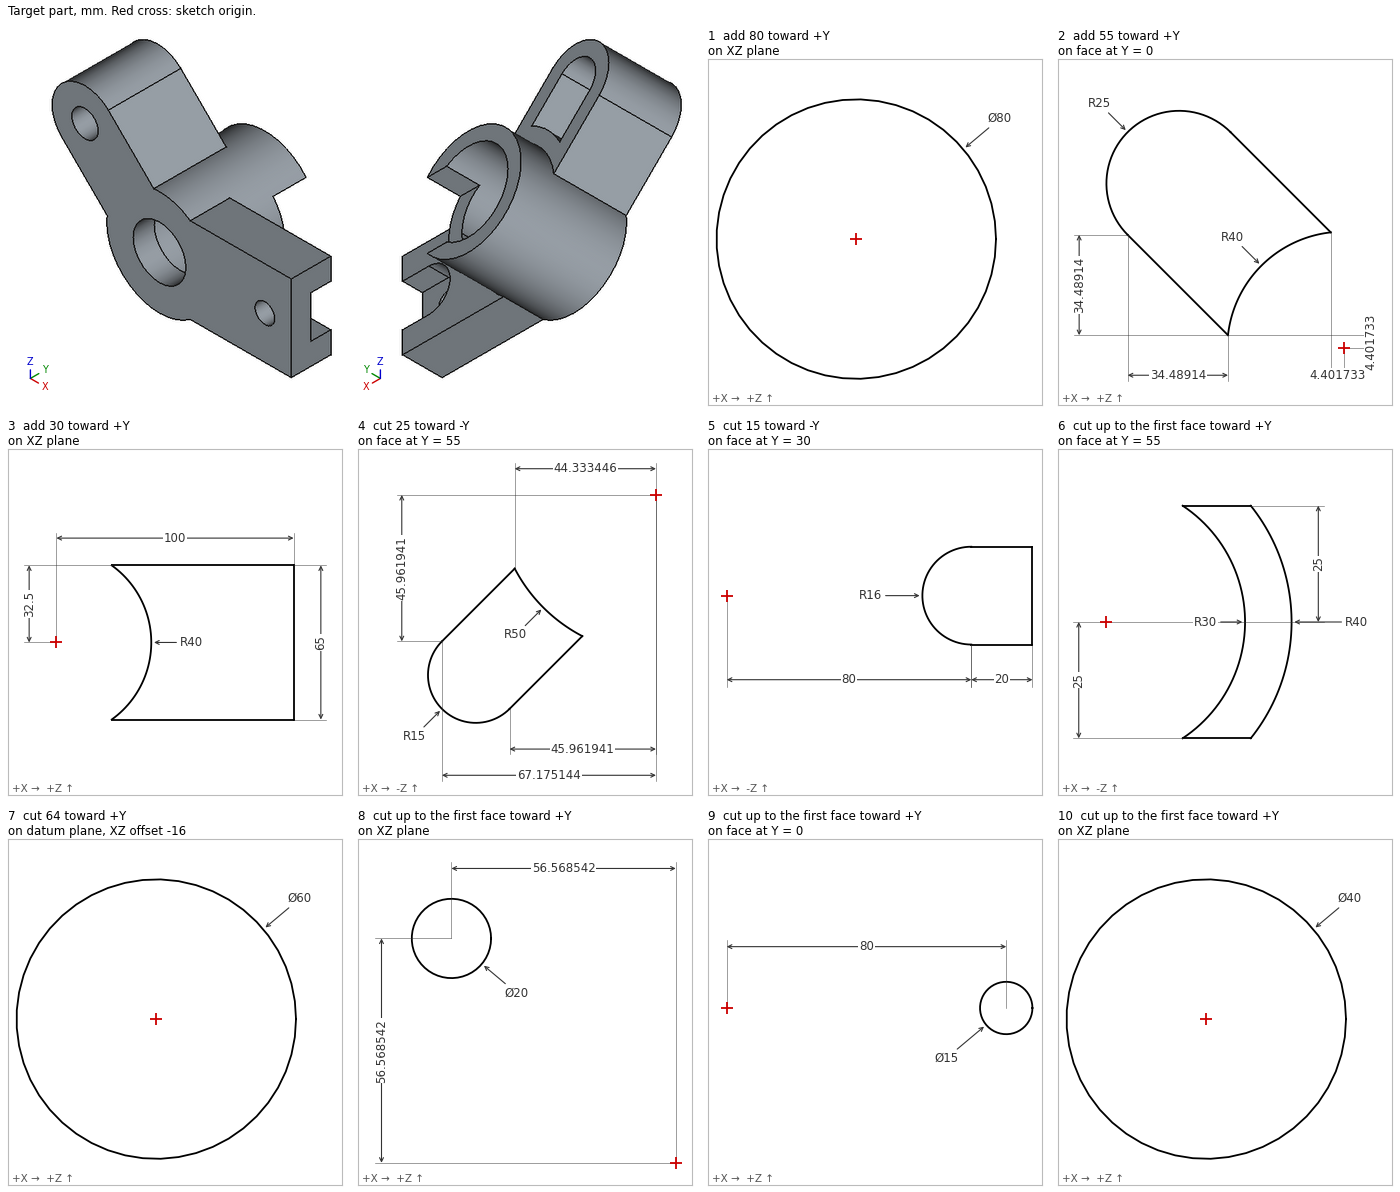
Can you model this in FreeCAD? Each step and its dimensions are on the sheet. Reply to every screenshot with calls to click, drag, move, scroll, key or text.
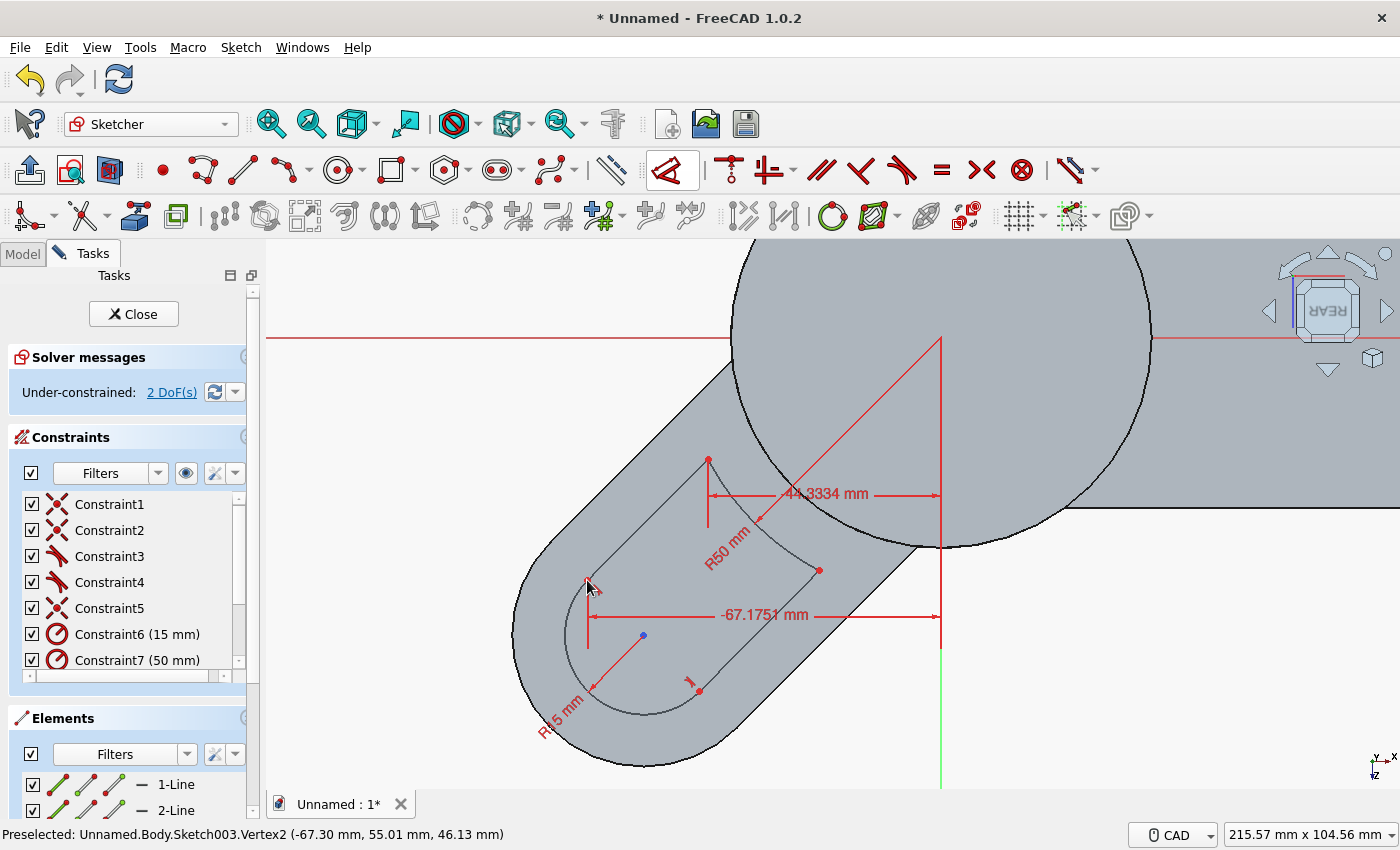
click(588, 580)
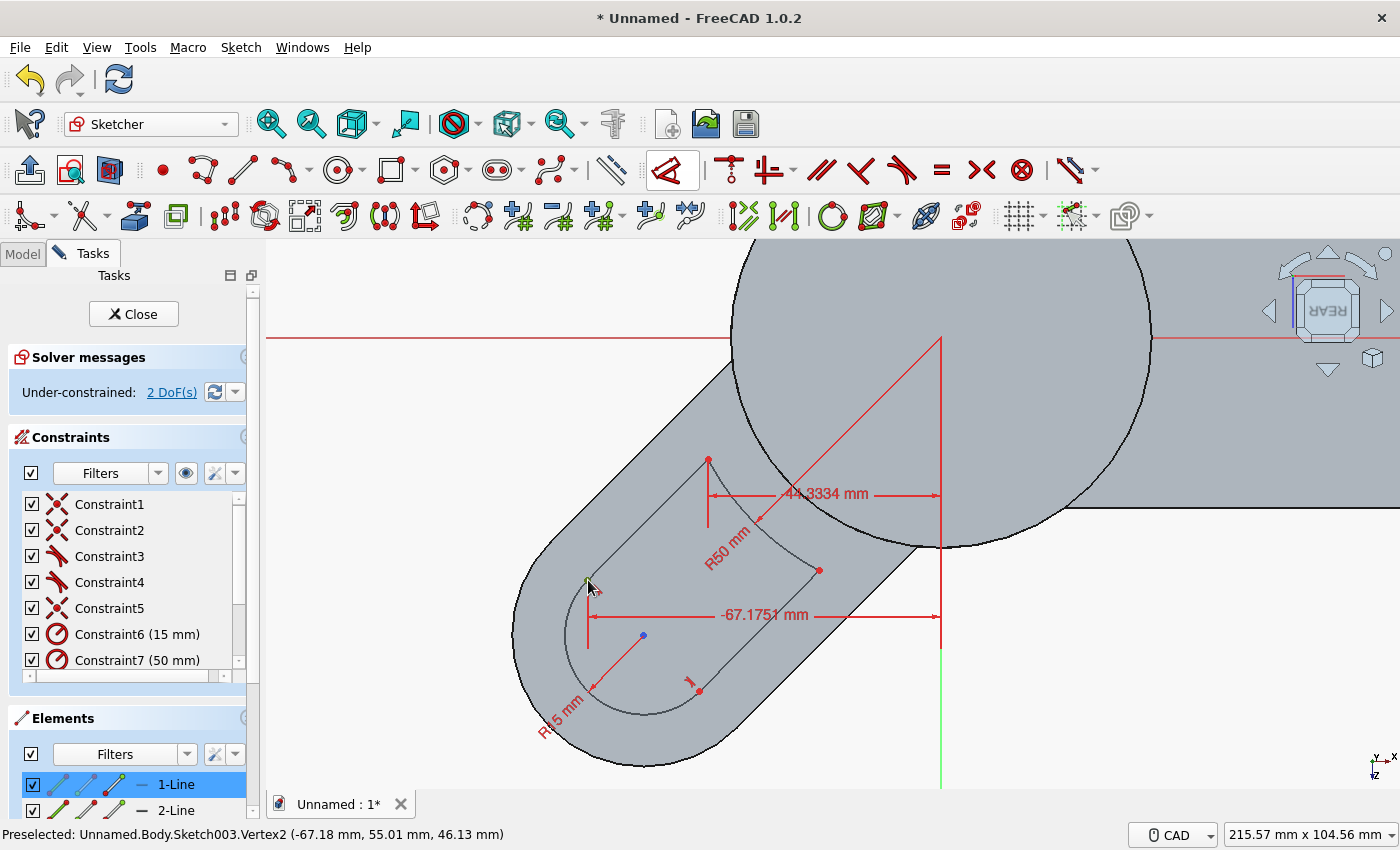
click(694, 170)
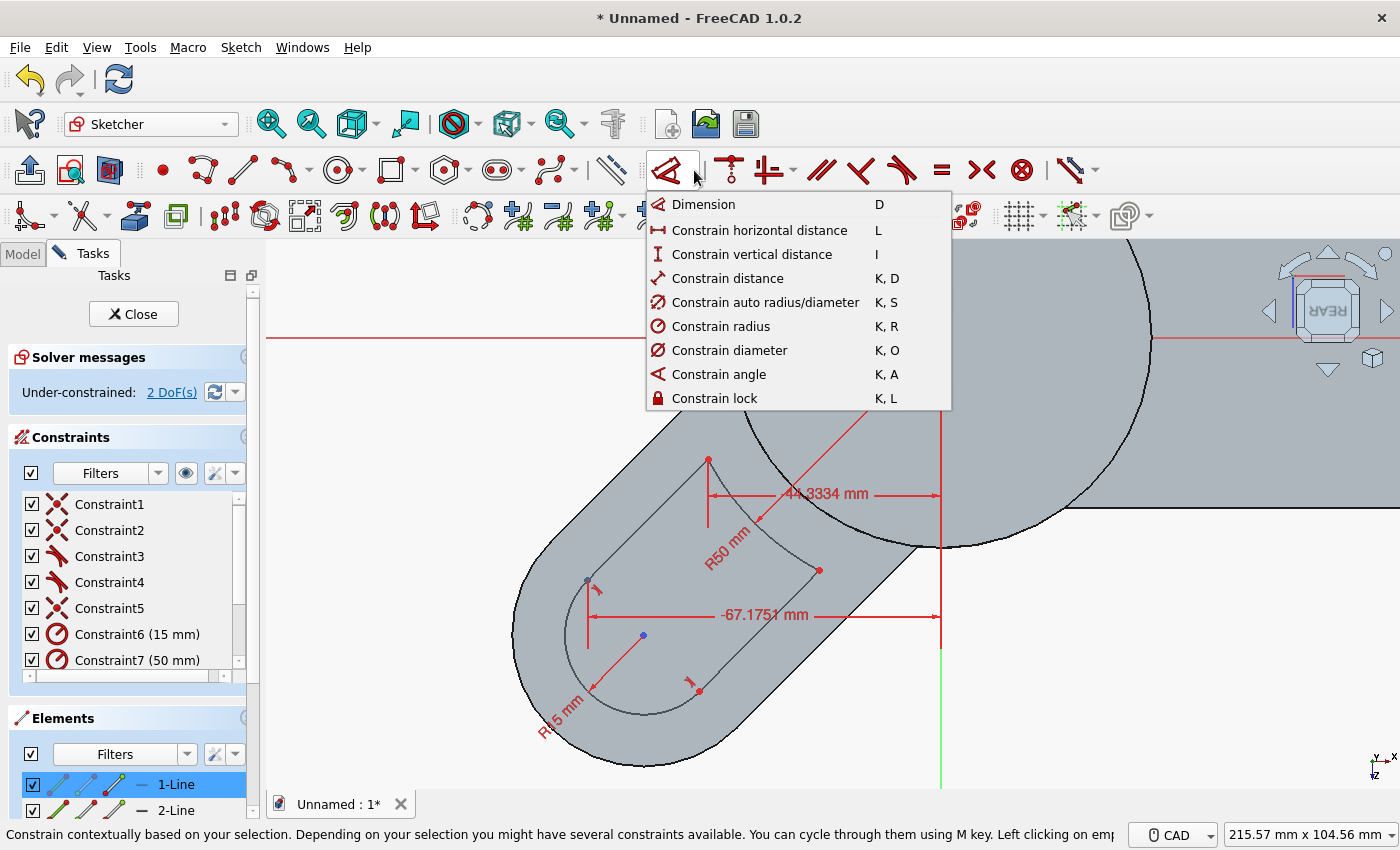
click(799, 254)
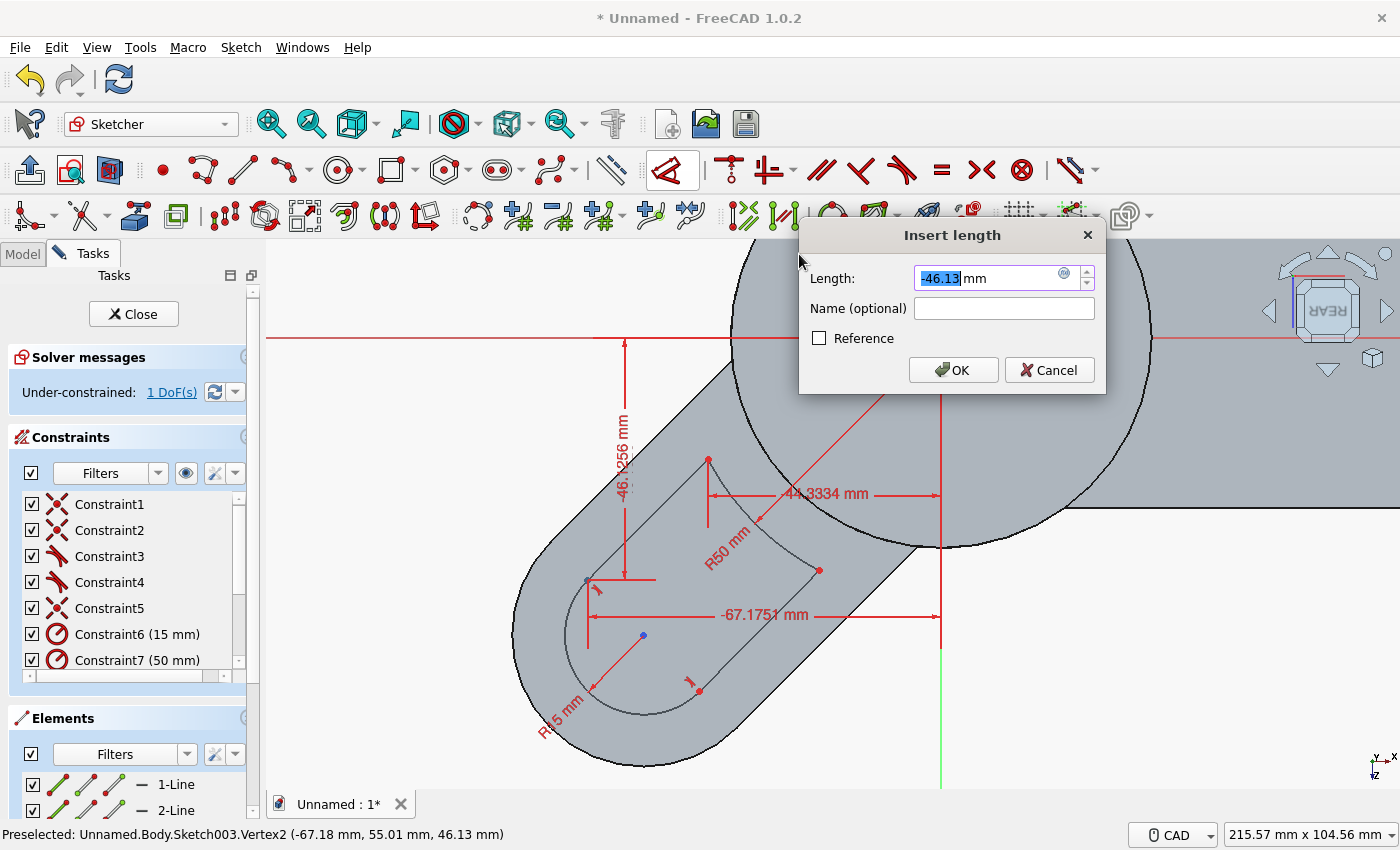
text(-45.961941)
key(Return)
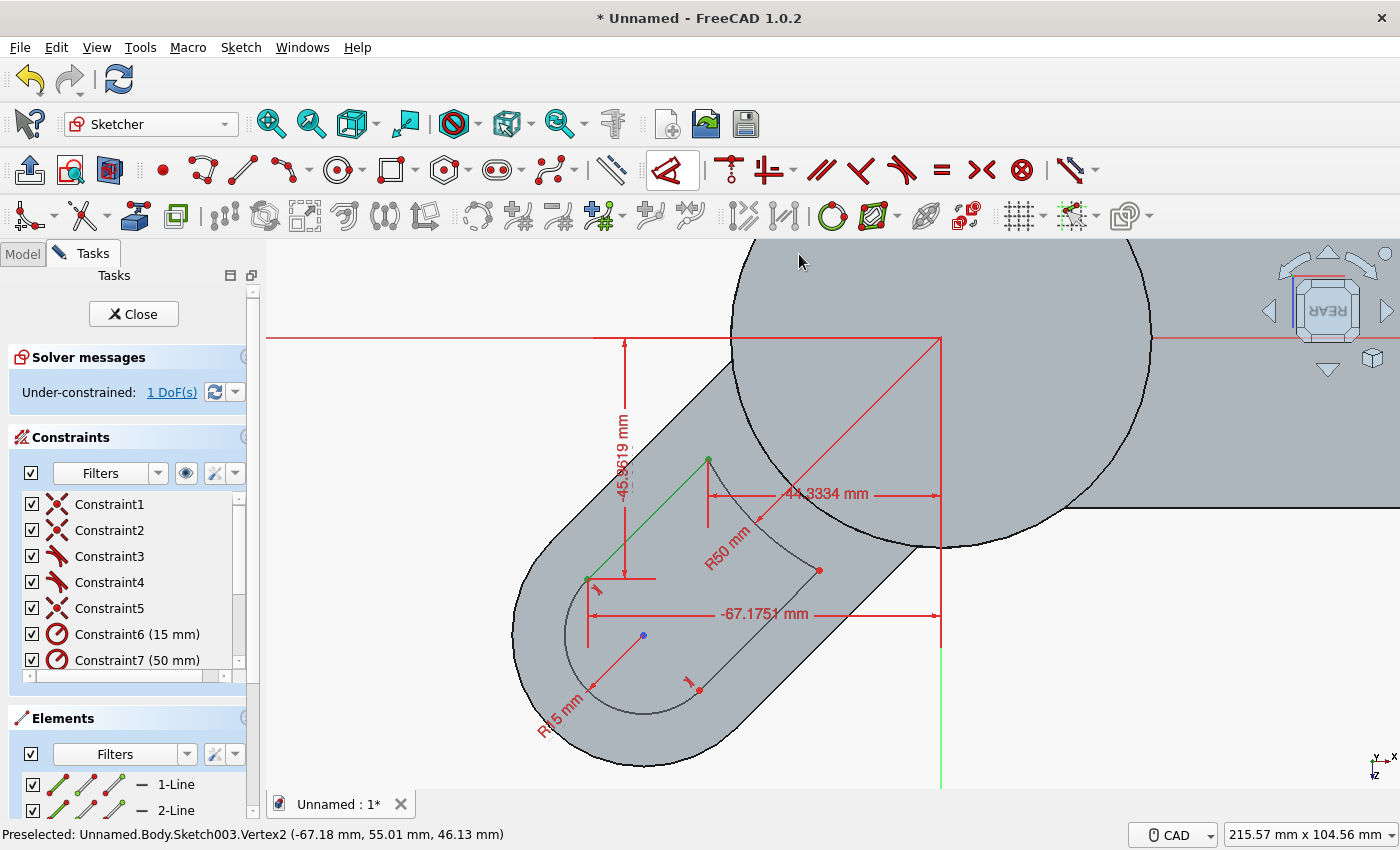
click(700, 691)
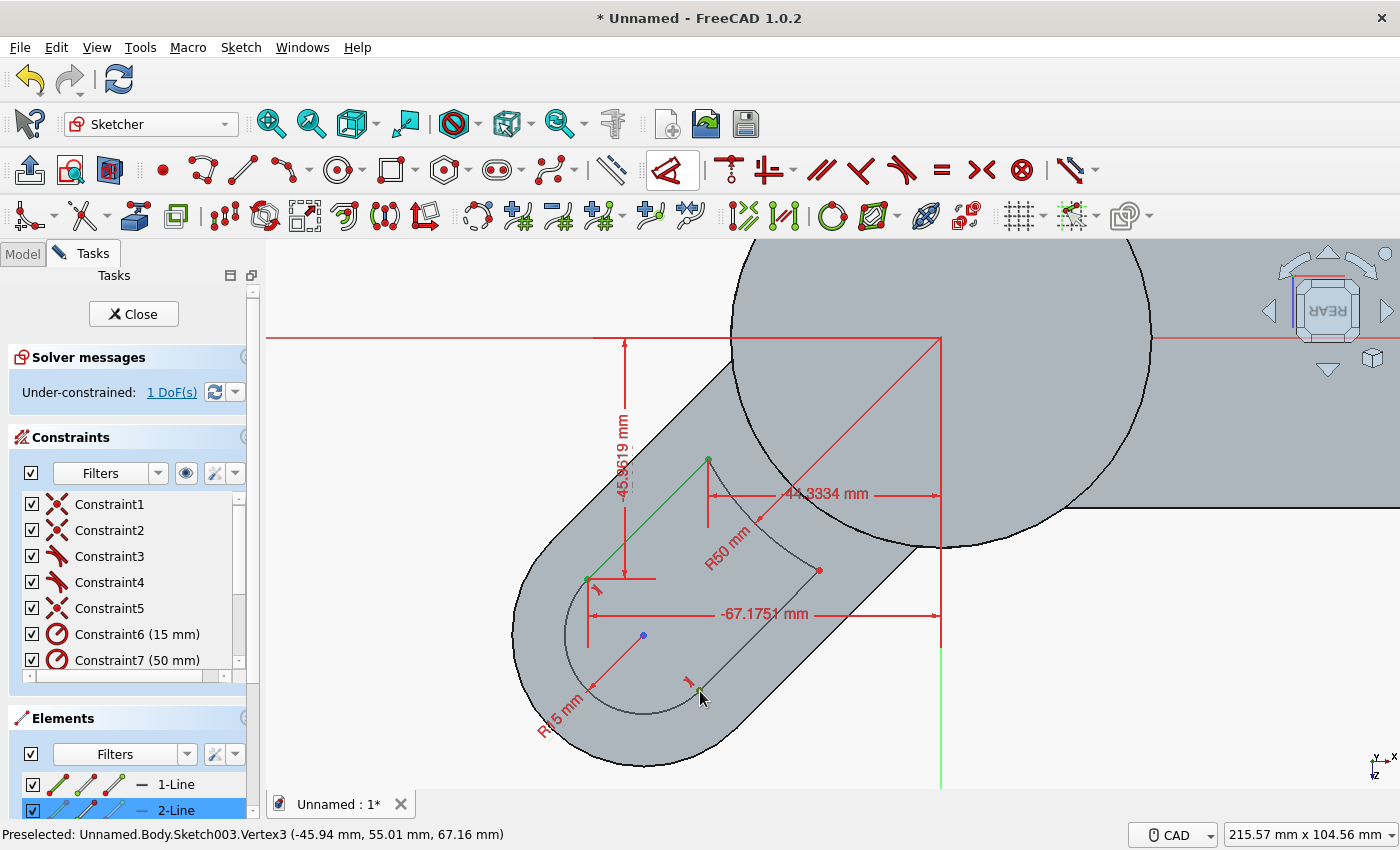
key(l)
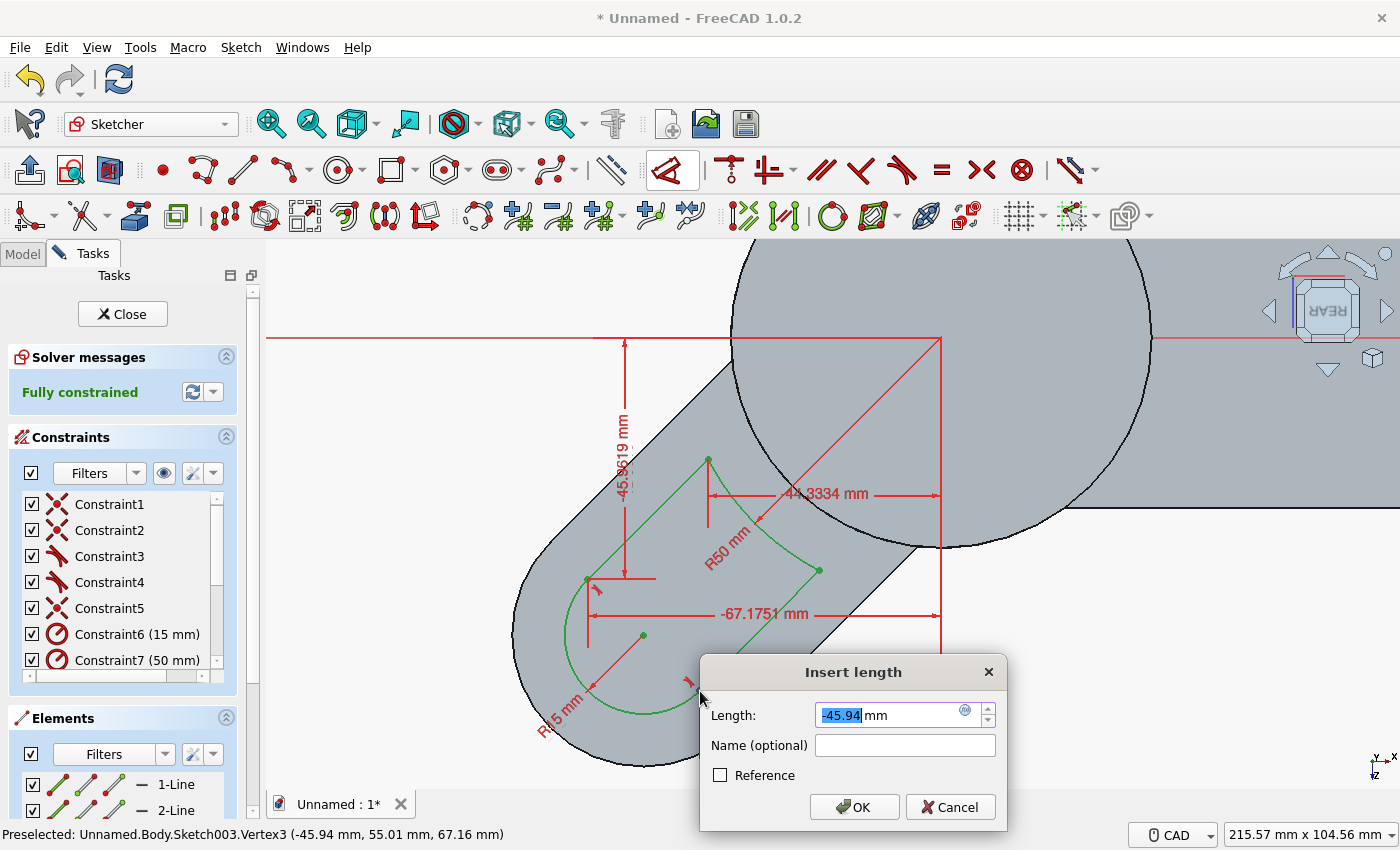
text(-45.961941)
key(Return)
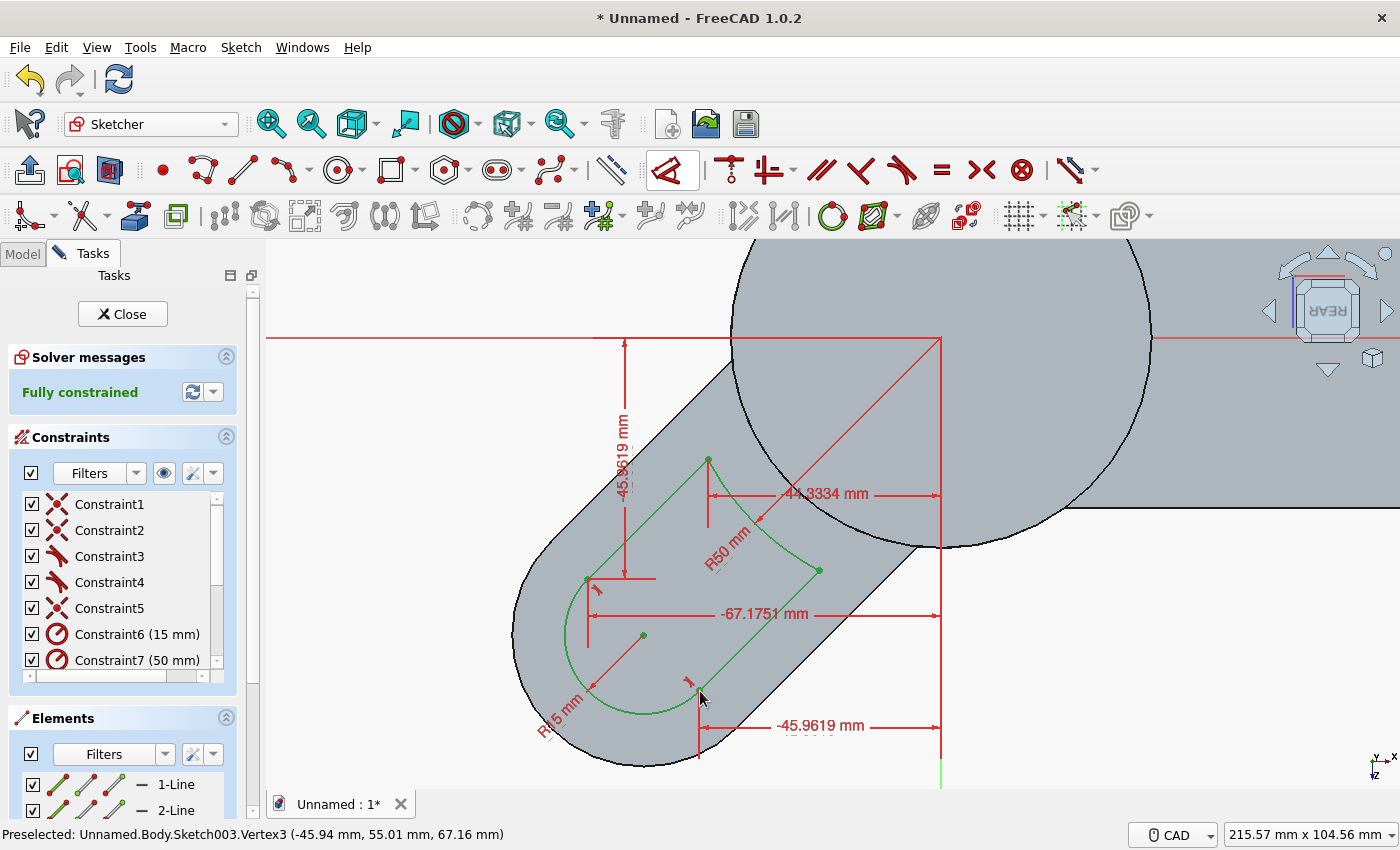
click(123, 314)